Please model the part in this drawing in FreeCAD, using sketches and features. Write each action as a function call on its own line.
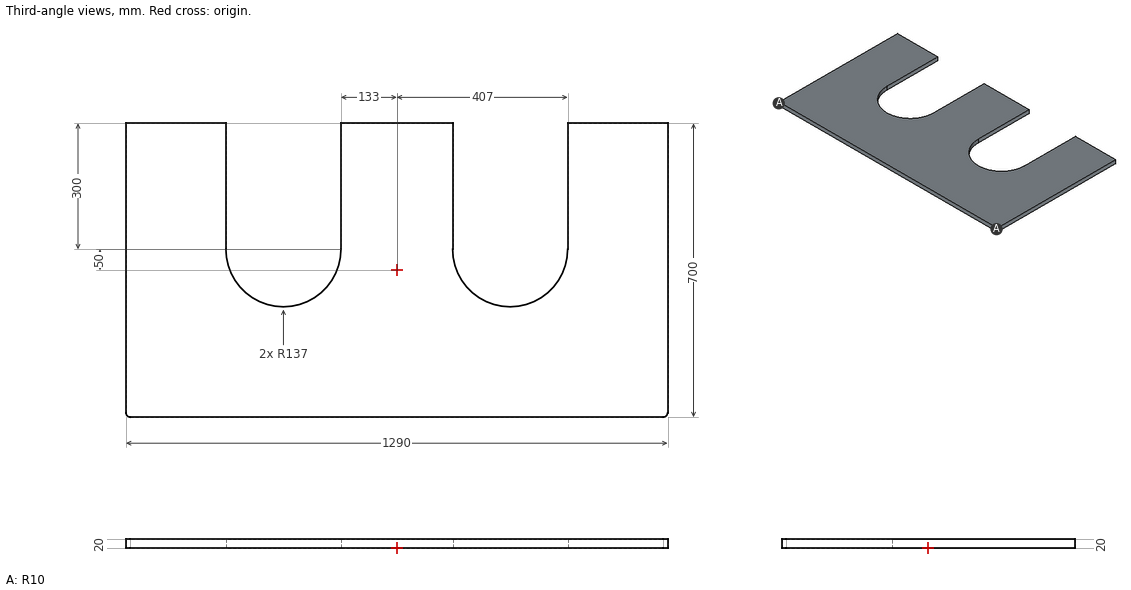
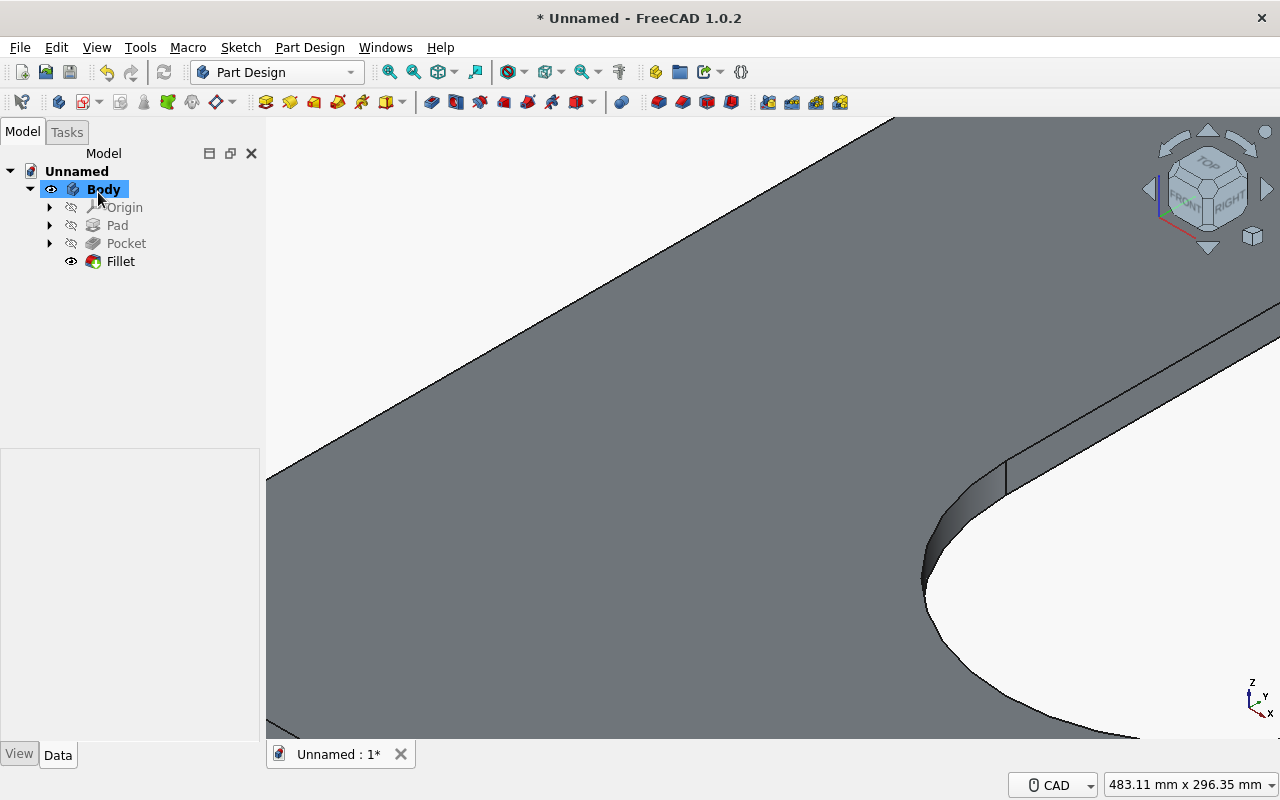
key(v)
key(f)